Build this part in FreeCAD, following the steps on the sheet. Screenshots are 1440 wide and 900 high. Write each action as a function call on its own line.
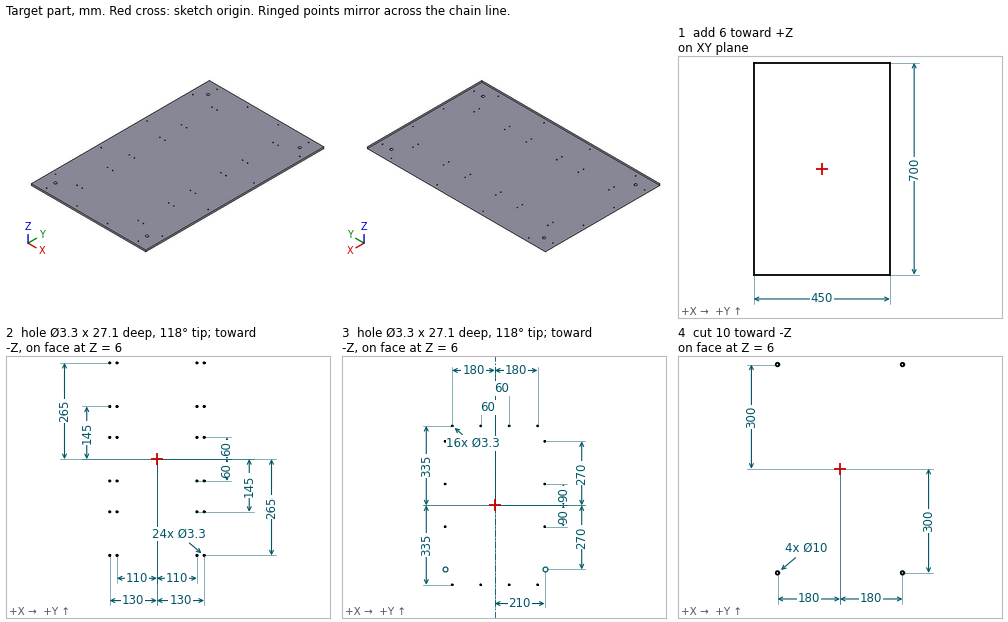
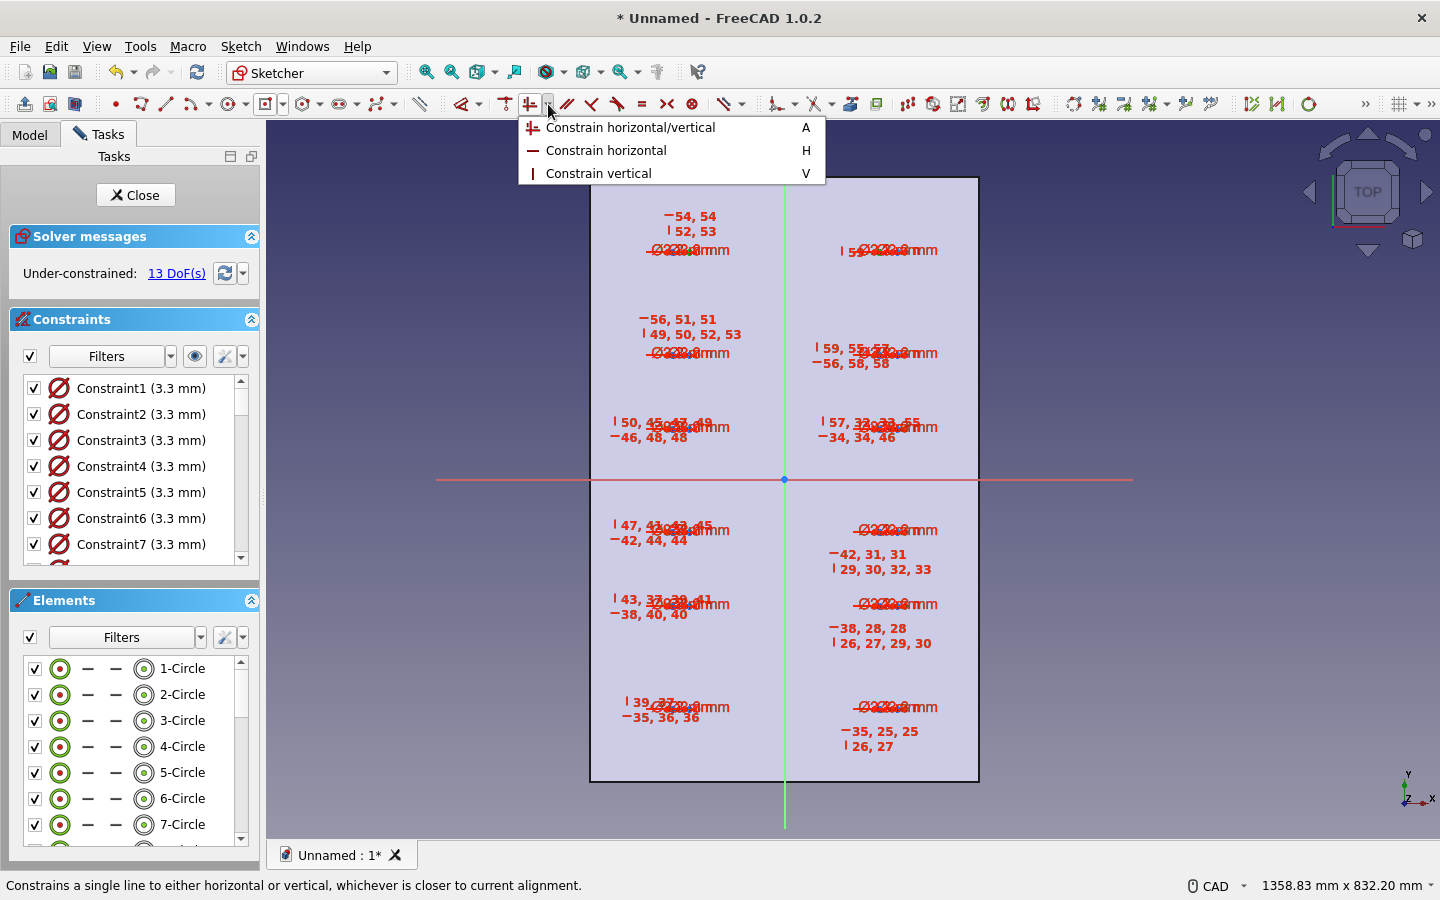
click(672, 150)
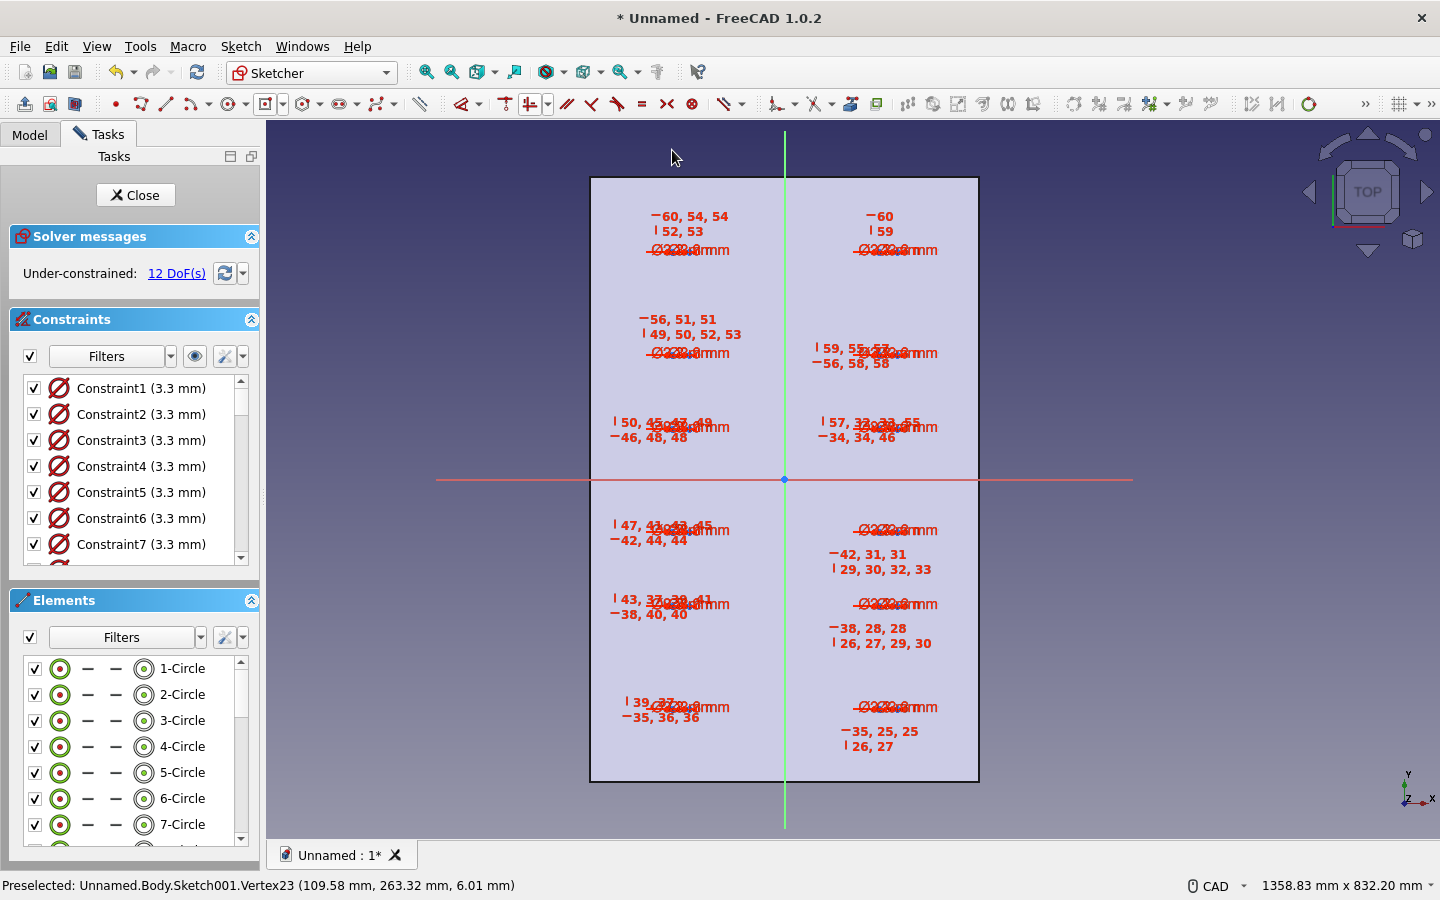
click(897, 355)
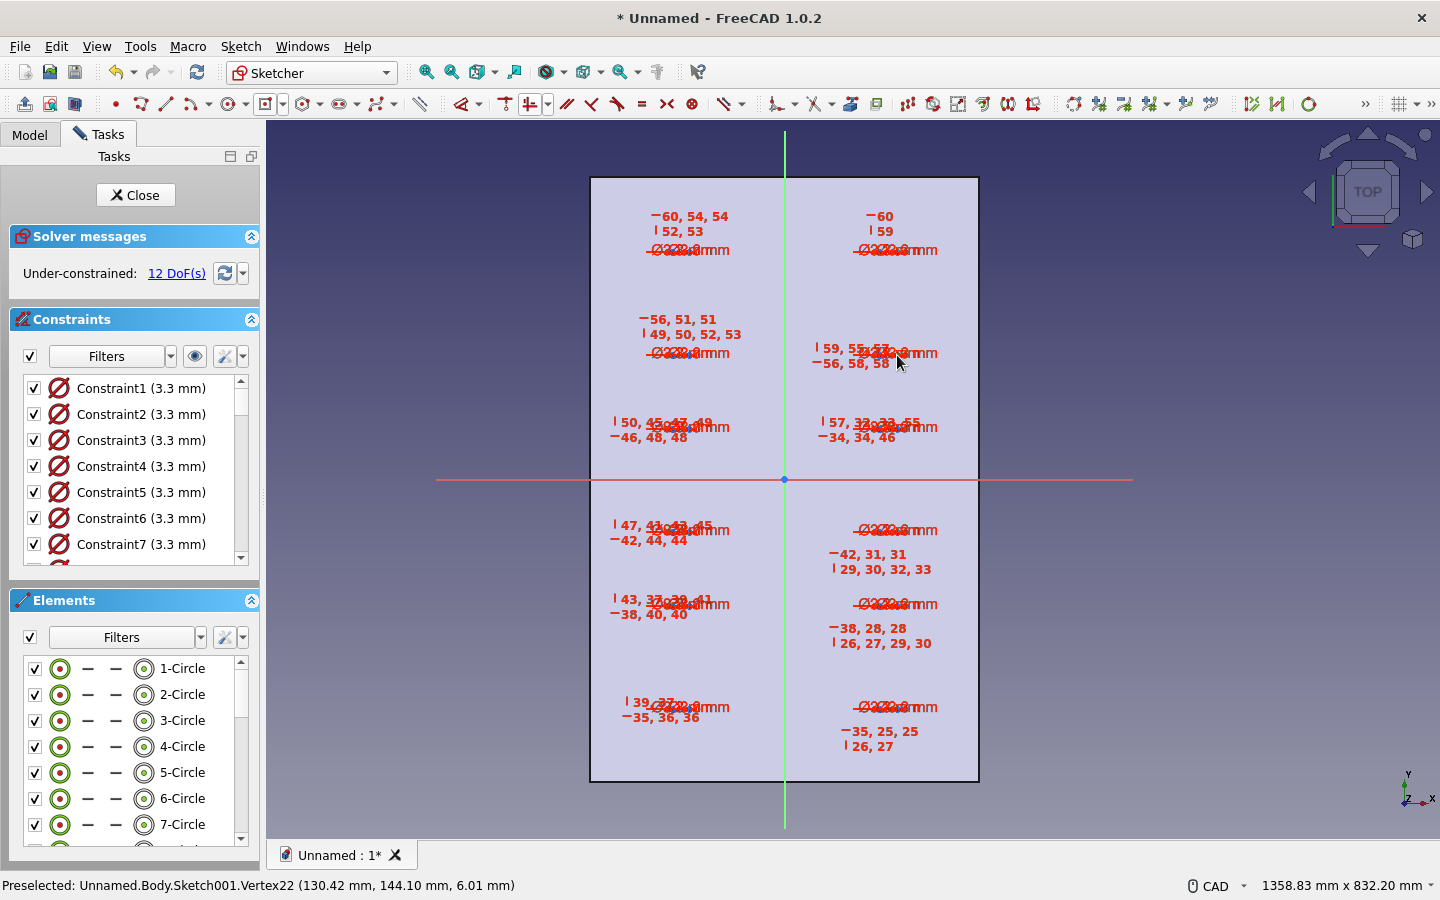
click(897, 252)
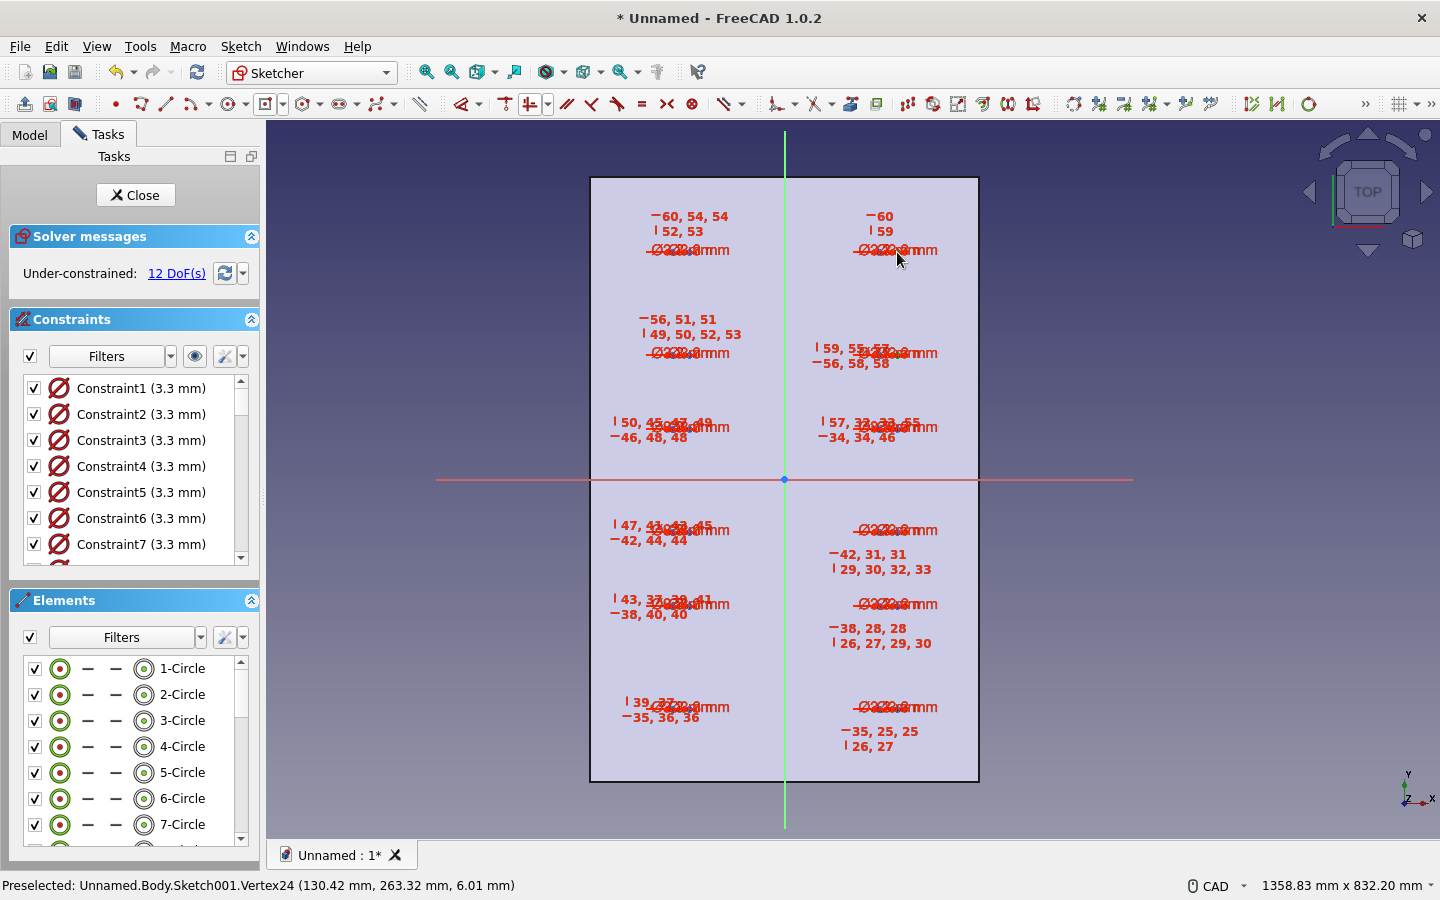
key(v)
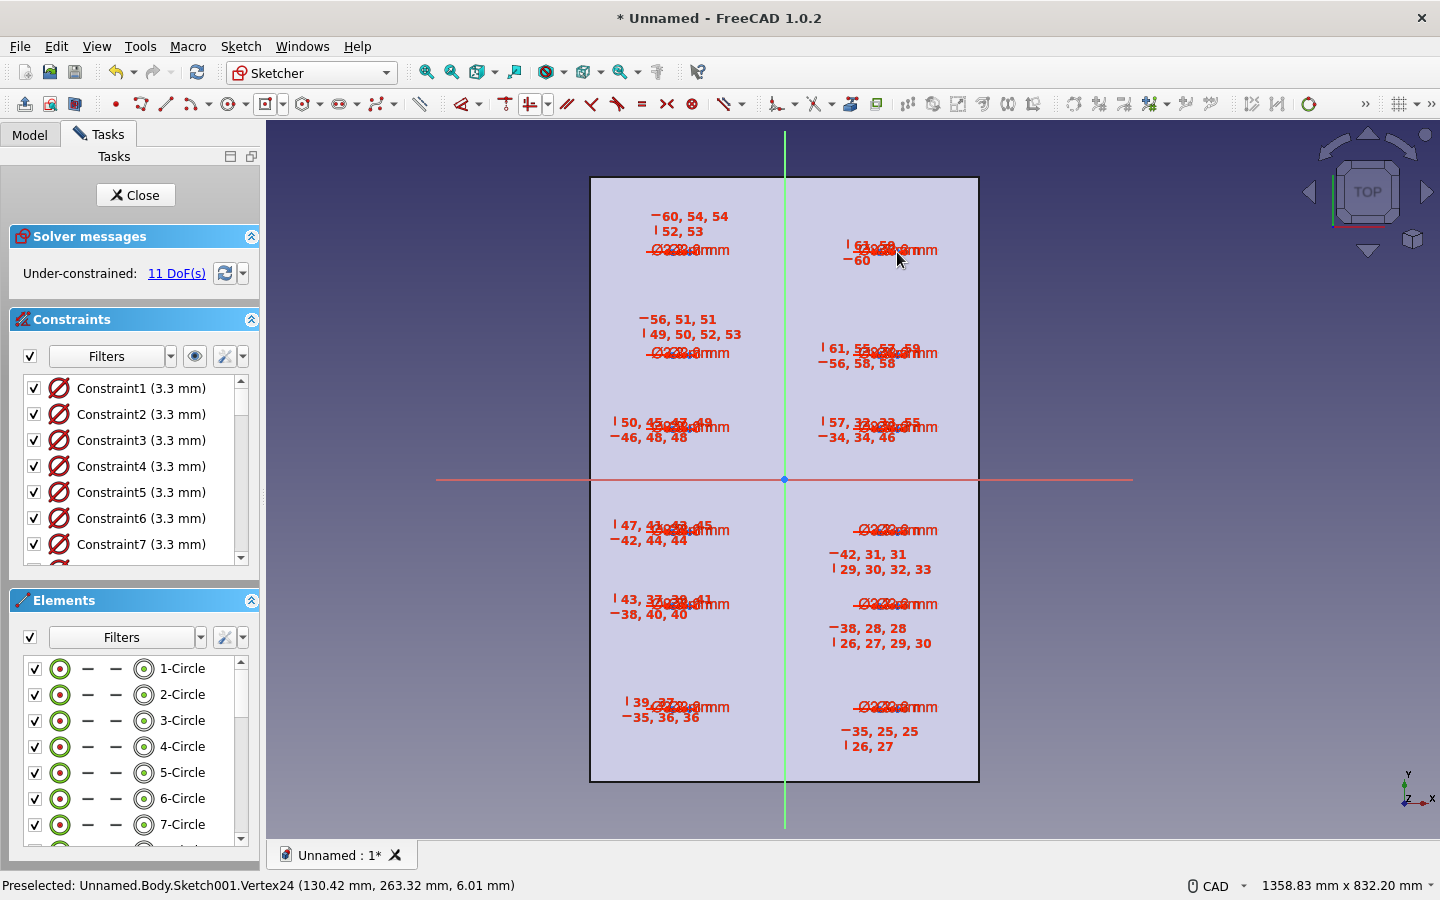
scroll(879, 252, up, 4)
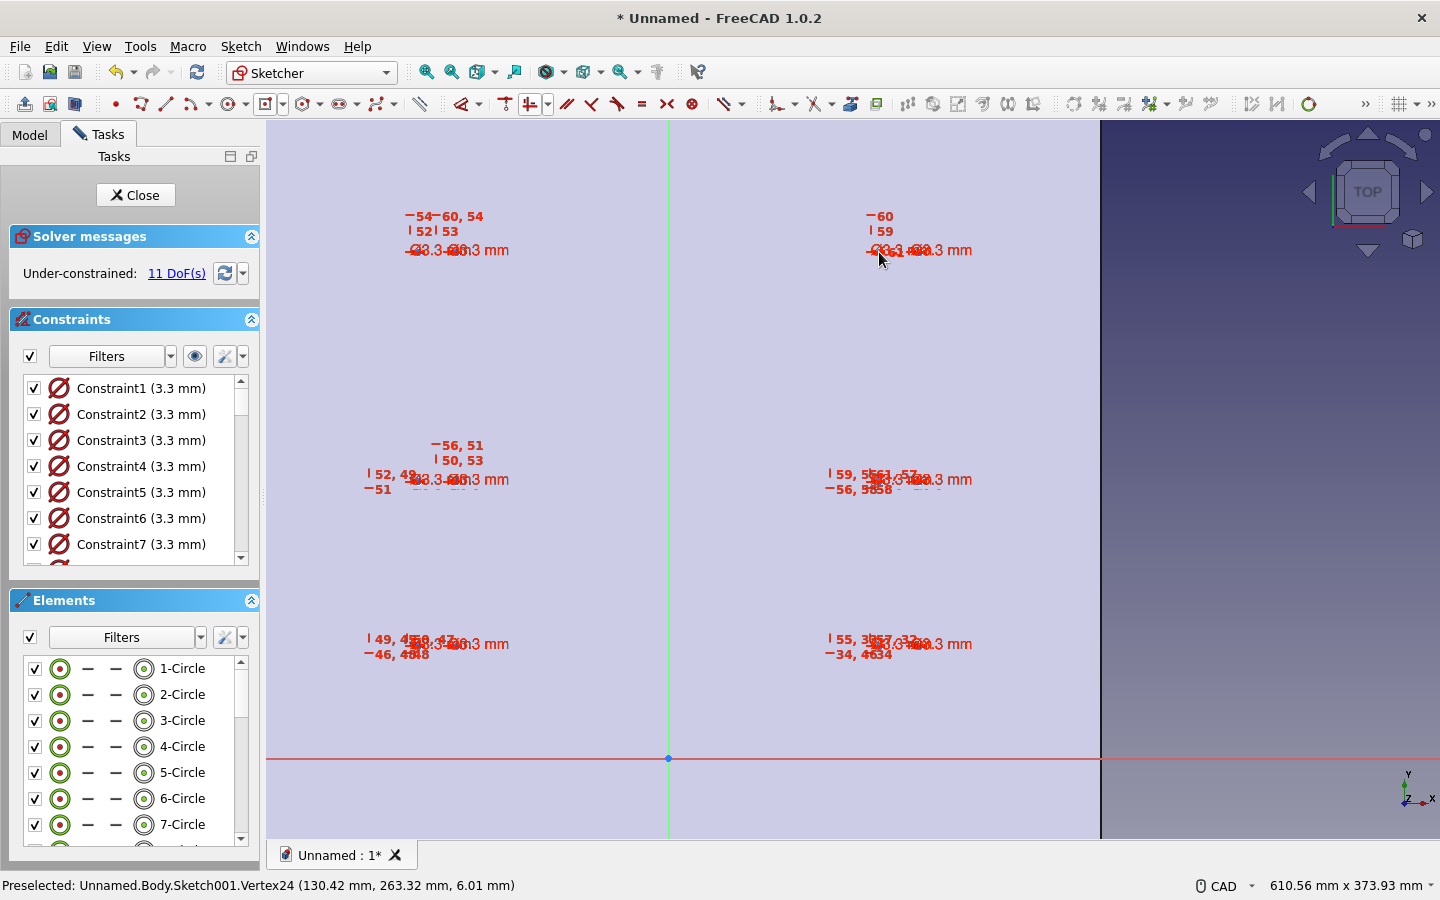
scroll(879, 252, up, 4)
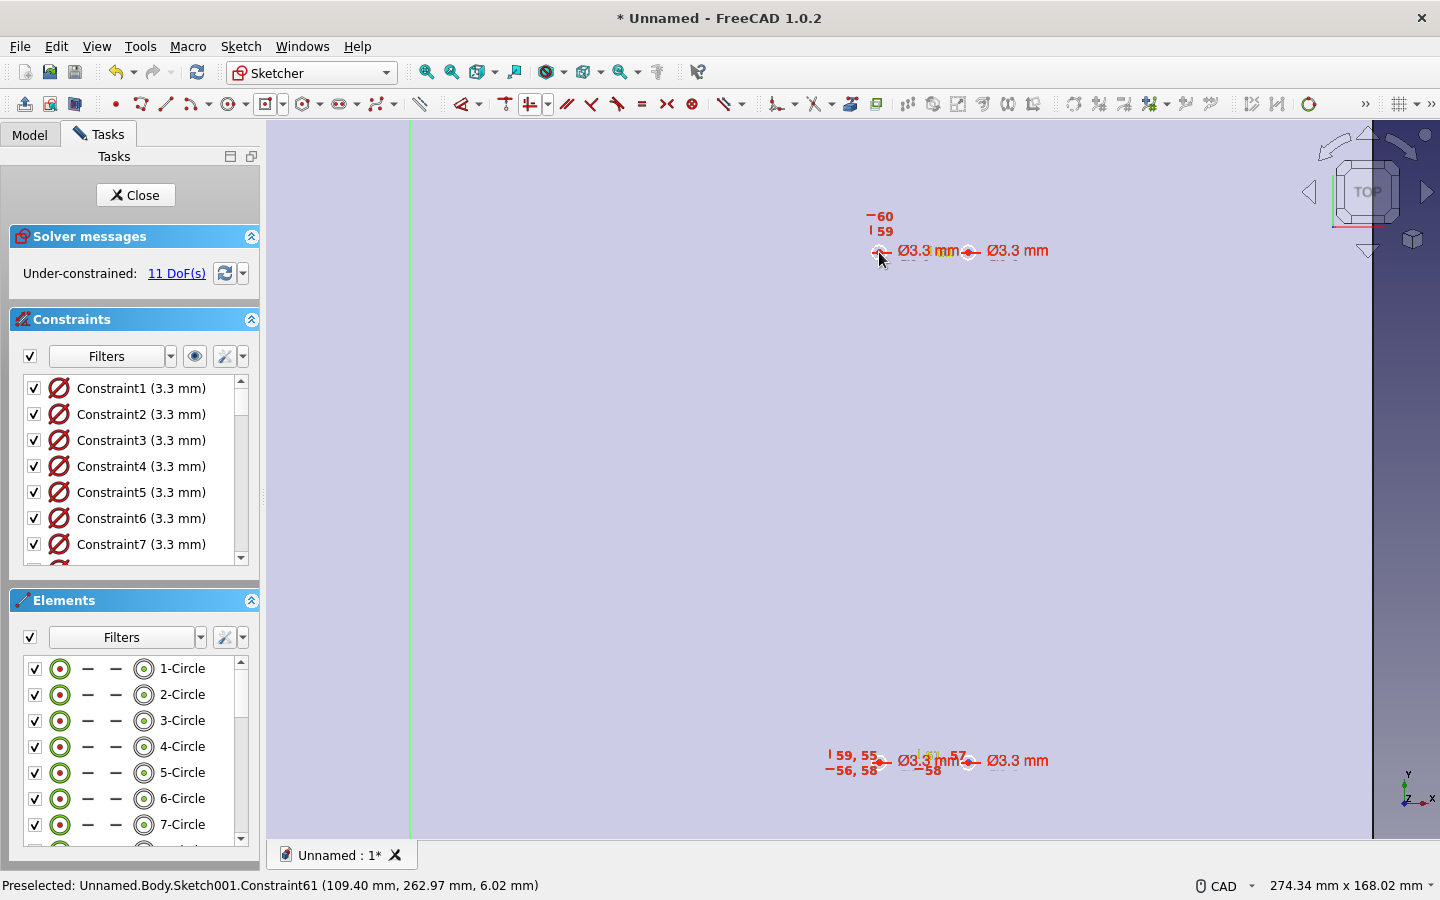
click(879, 253)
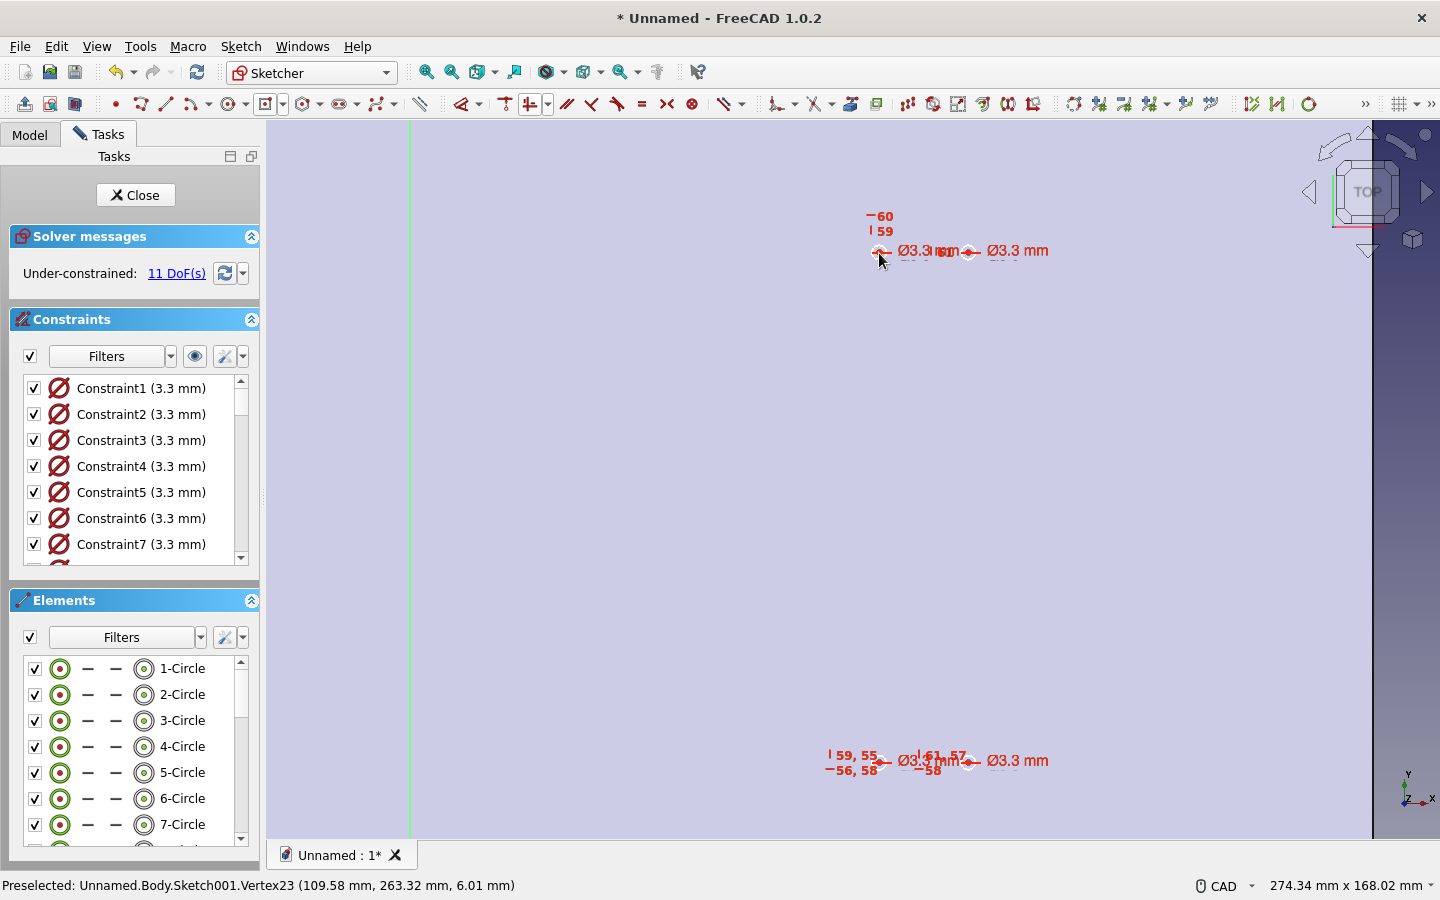
scroll(879, 252, down, 8)